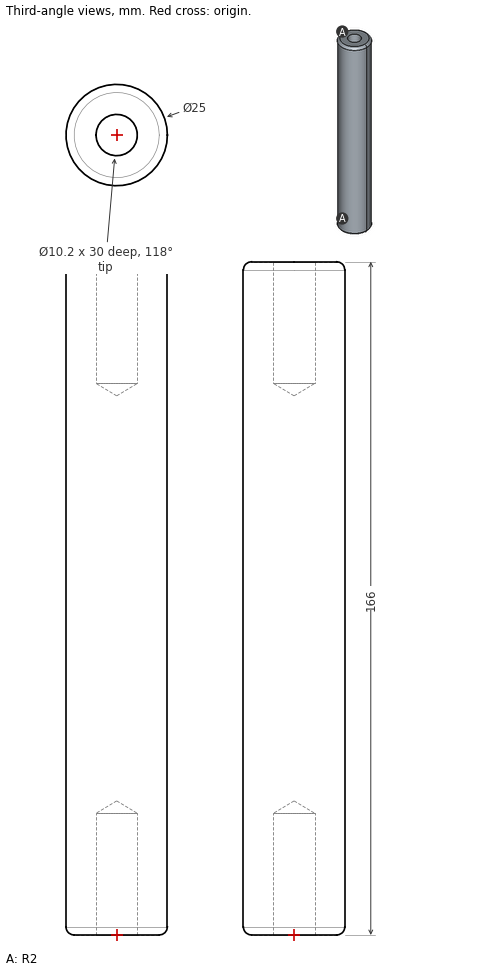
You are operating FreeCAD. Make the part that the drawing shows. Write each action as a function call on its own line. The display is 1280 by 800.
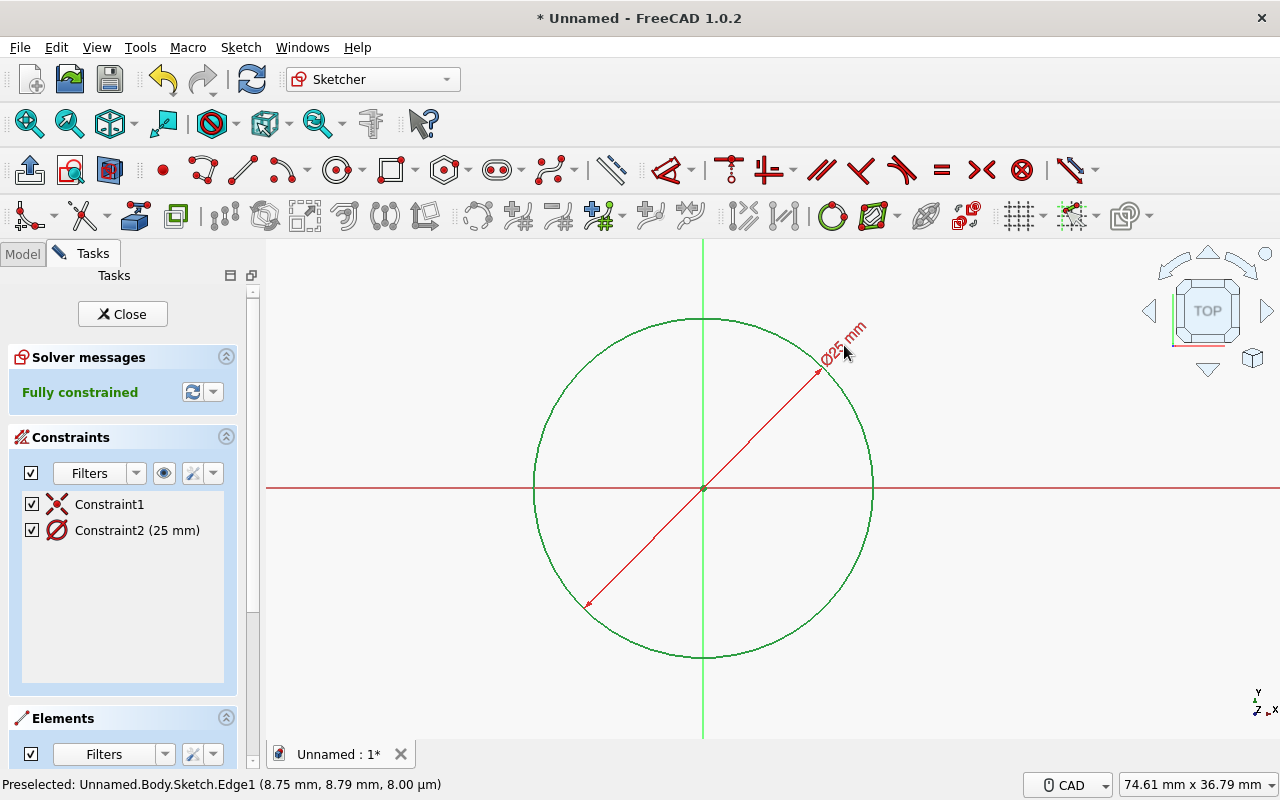
click(123, 314)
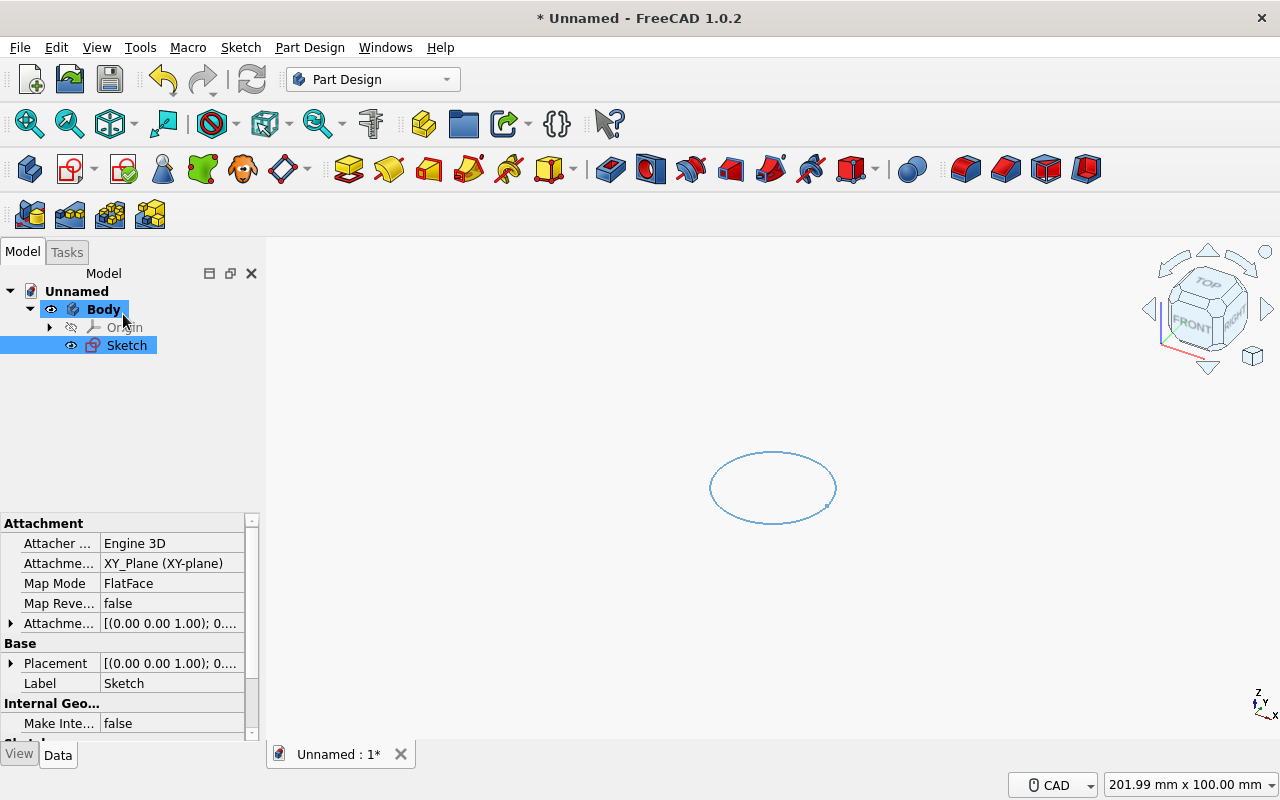
click(350, 170)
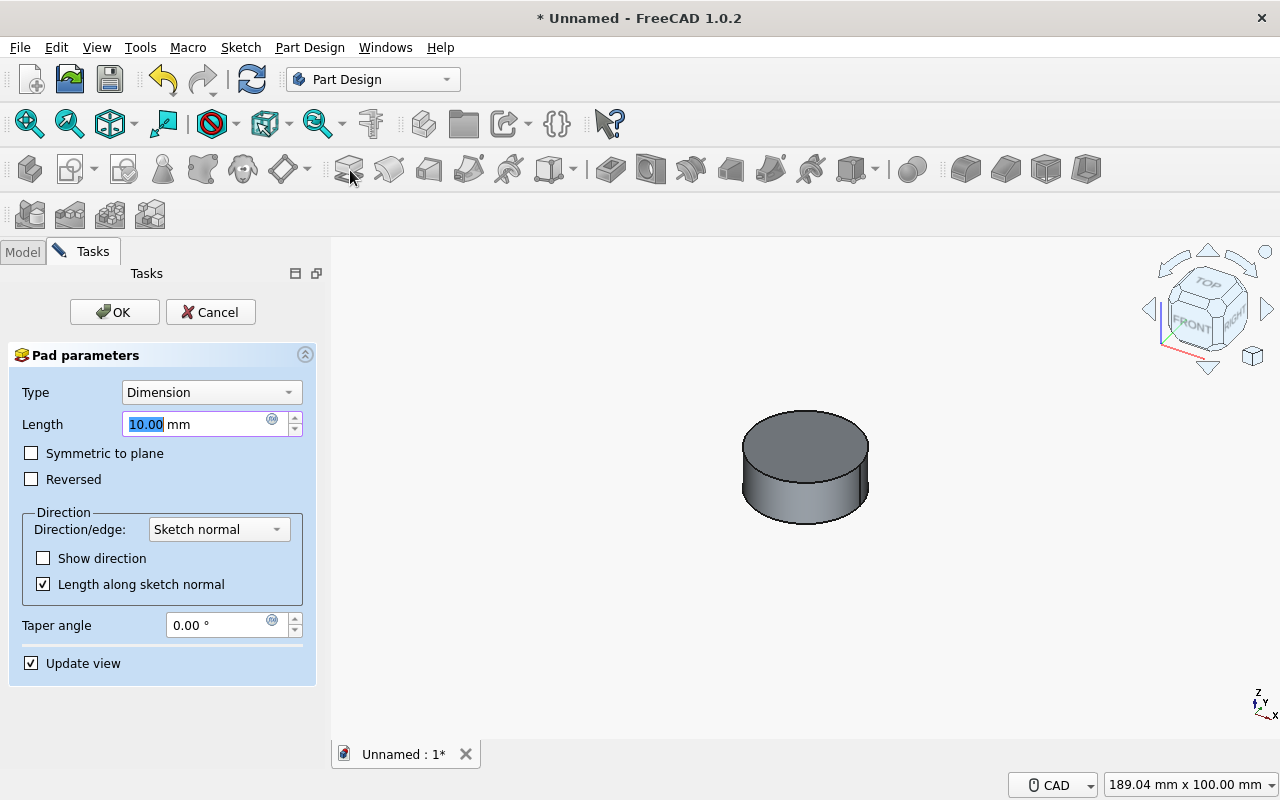
text(166)
key(Tab)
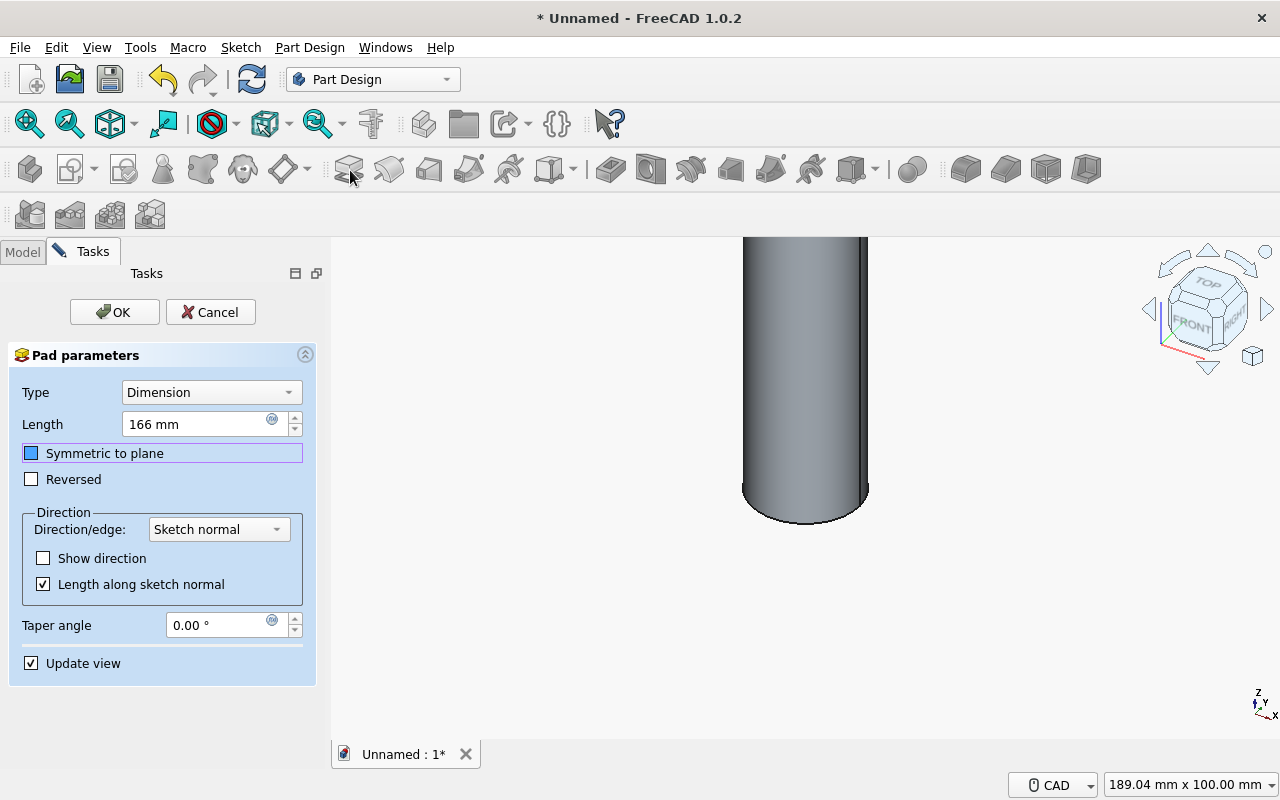
click(115, 312)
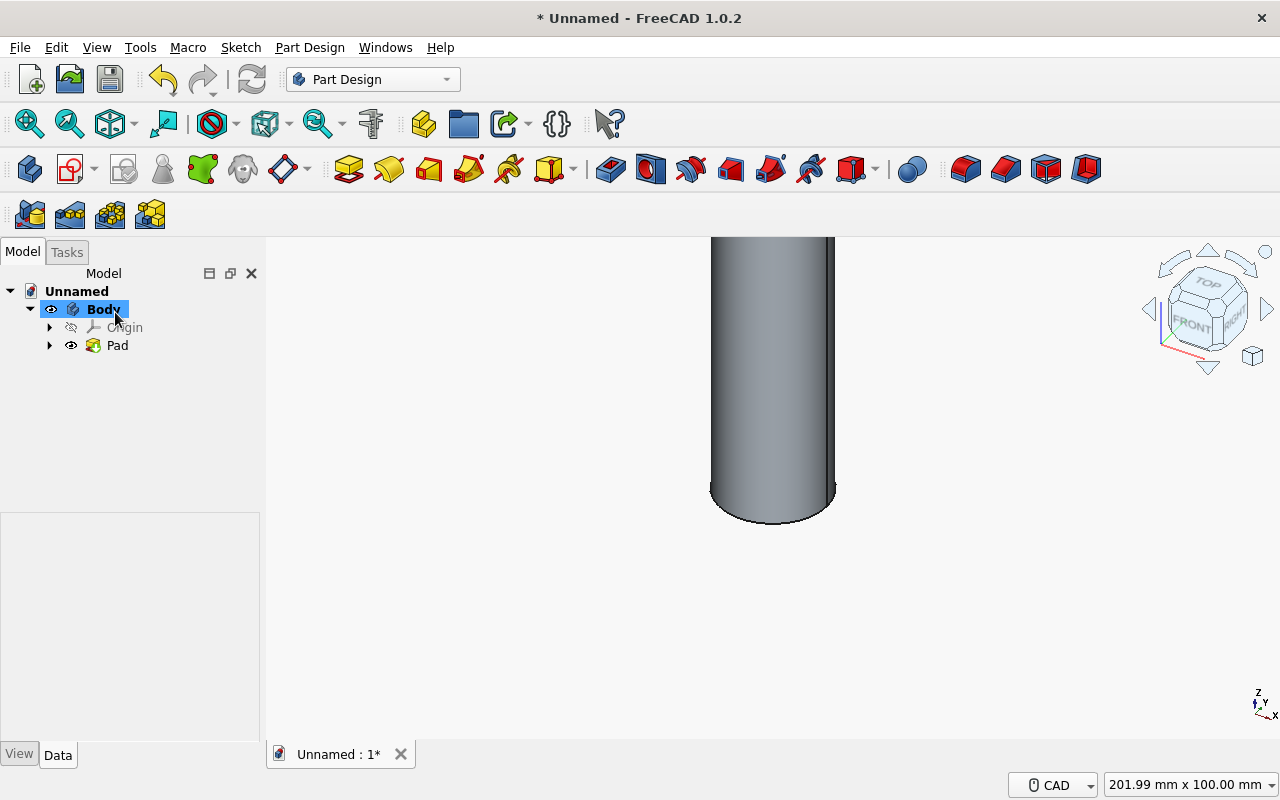
click(30, 124)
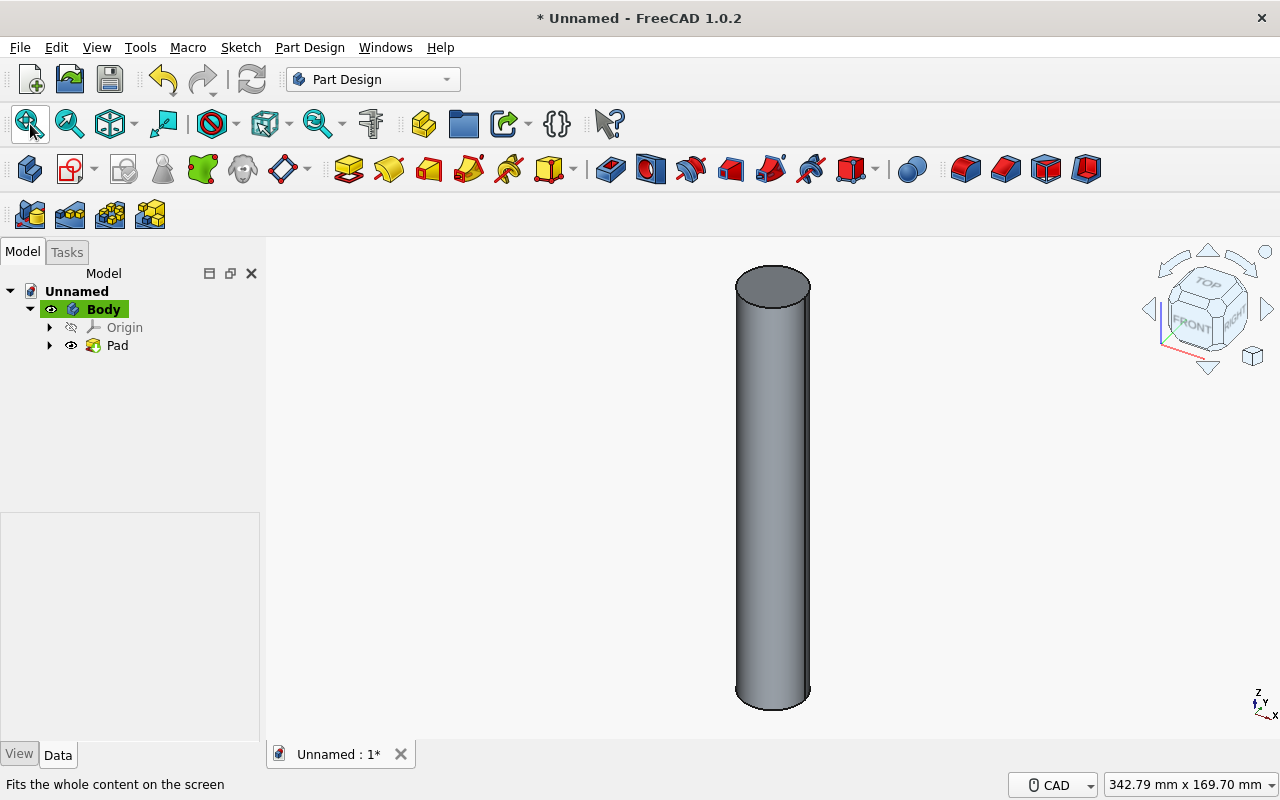
click(736, 288)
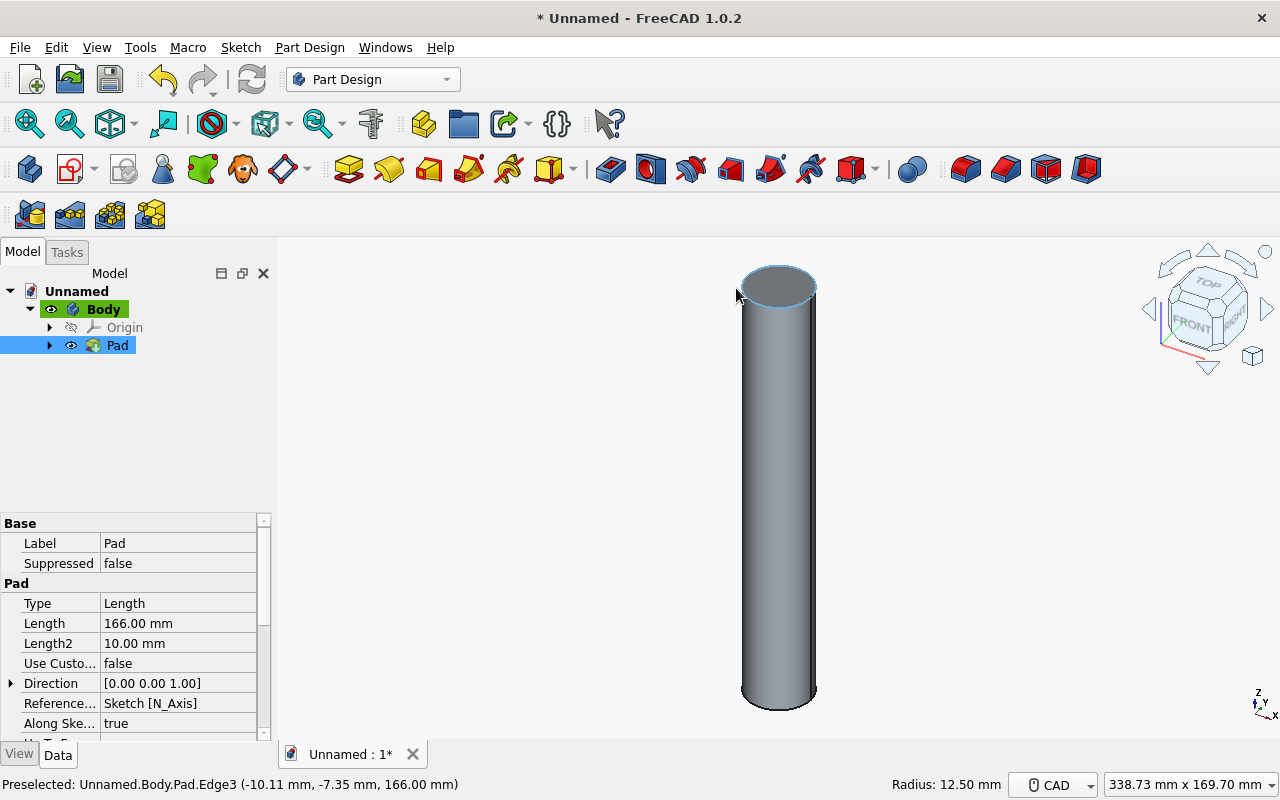
key(0)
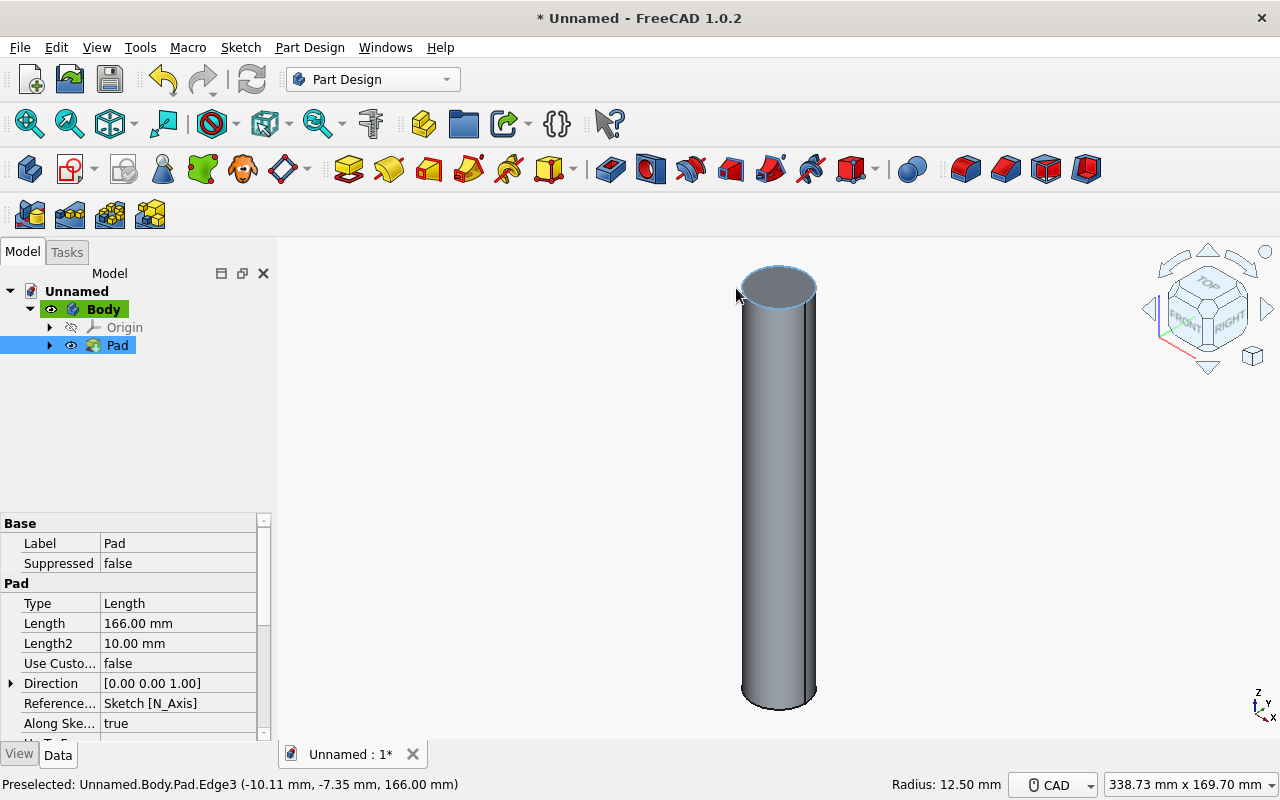
key(2)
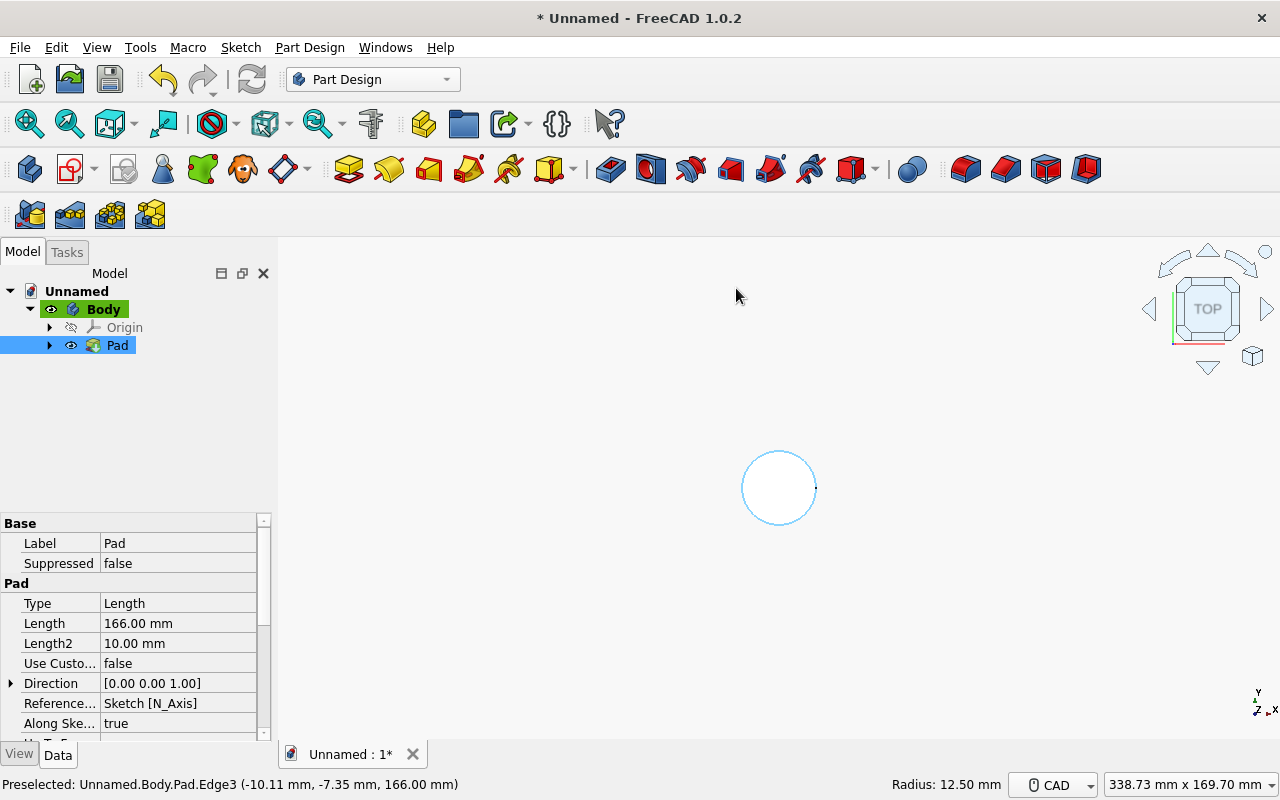
click(30, 124)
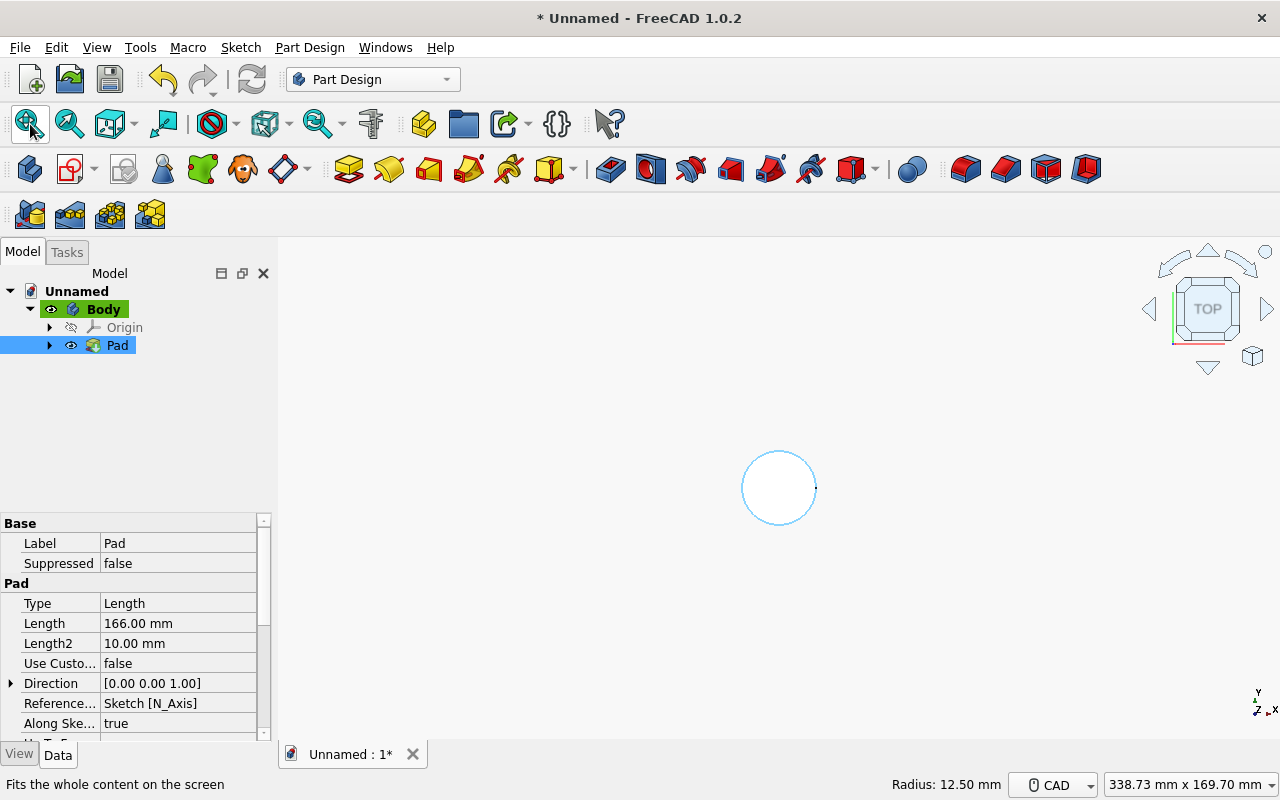
key(1)